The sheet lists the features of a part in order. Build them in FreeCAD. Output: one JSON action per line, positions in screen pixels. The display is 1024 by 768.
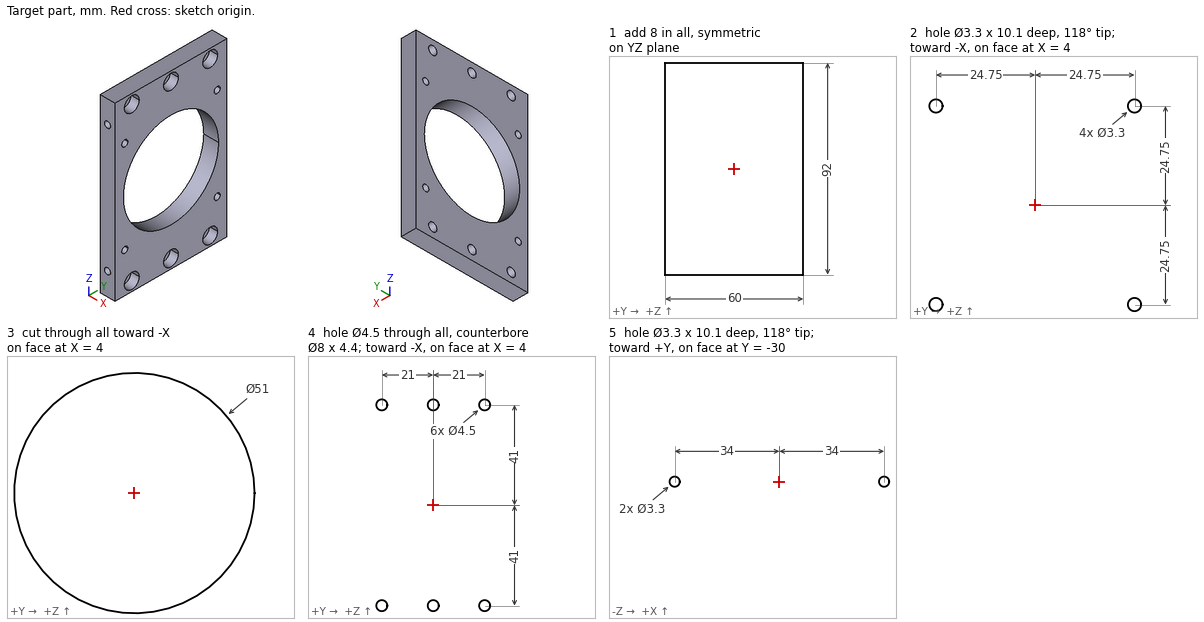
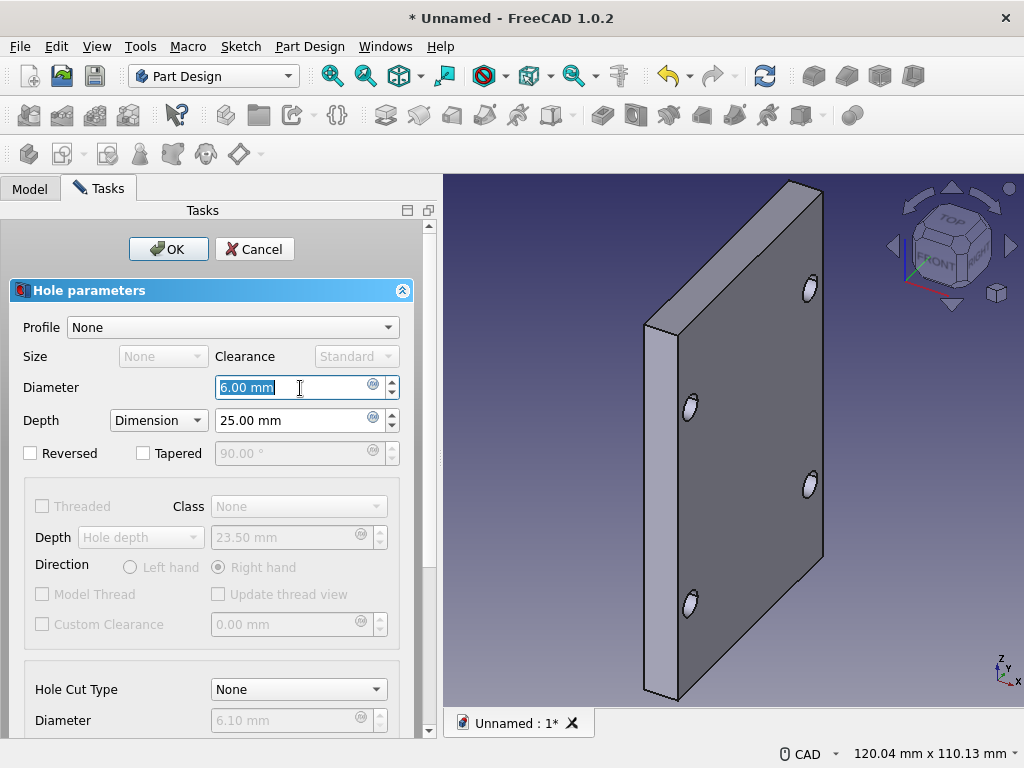
{"action": "type", "text": "3.3"}
{"action": "key", "text": "Tab"}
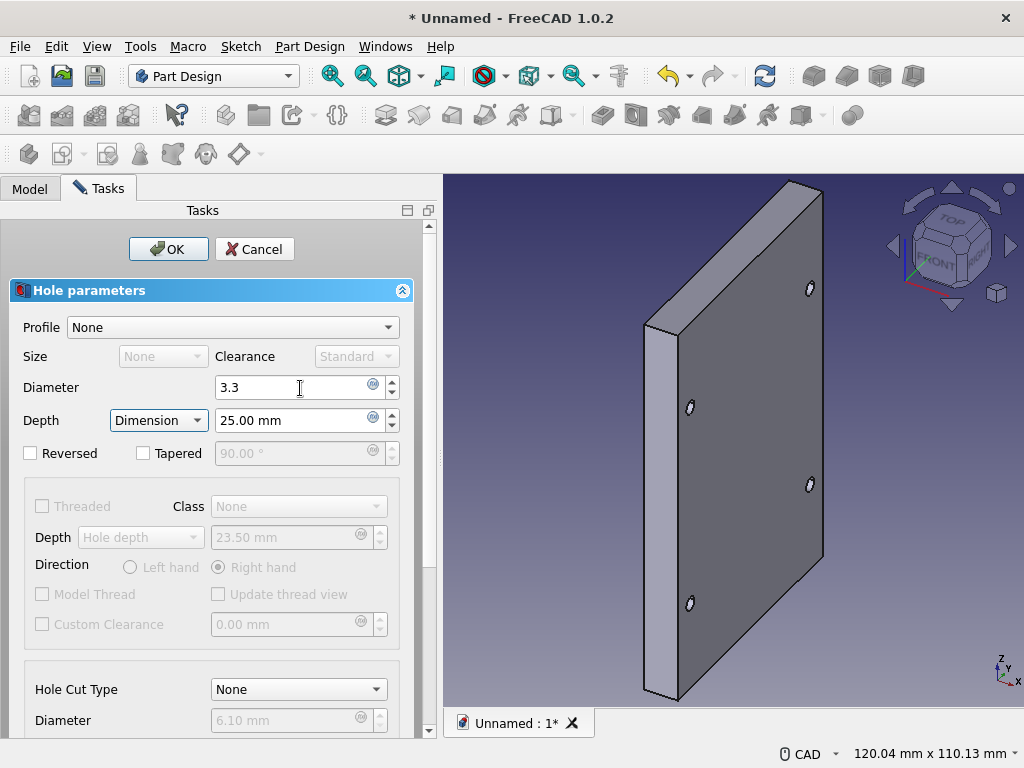
{"action": "triple_click", "coordinate": [300, 420]}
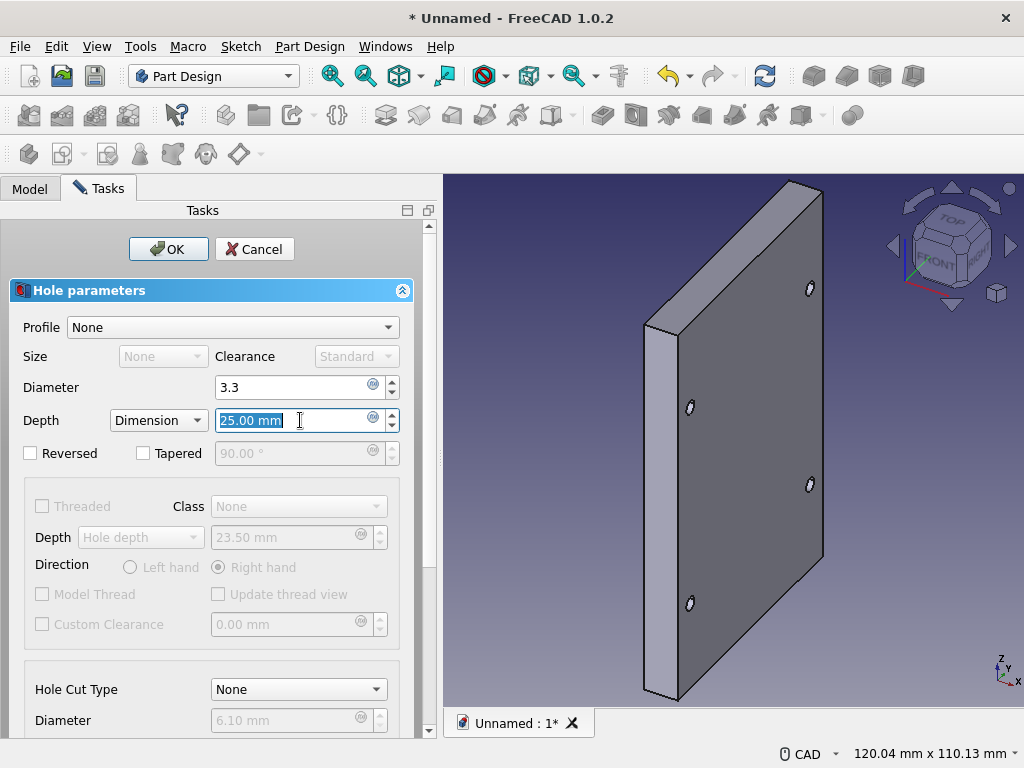
{"action": "type", "text": "10.1"}
{"action": "key", "text": "Tab"}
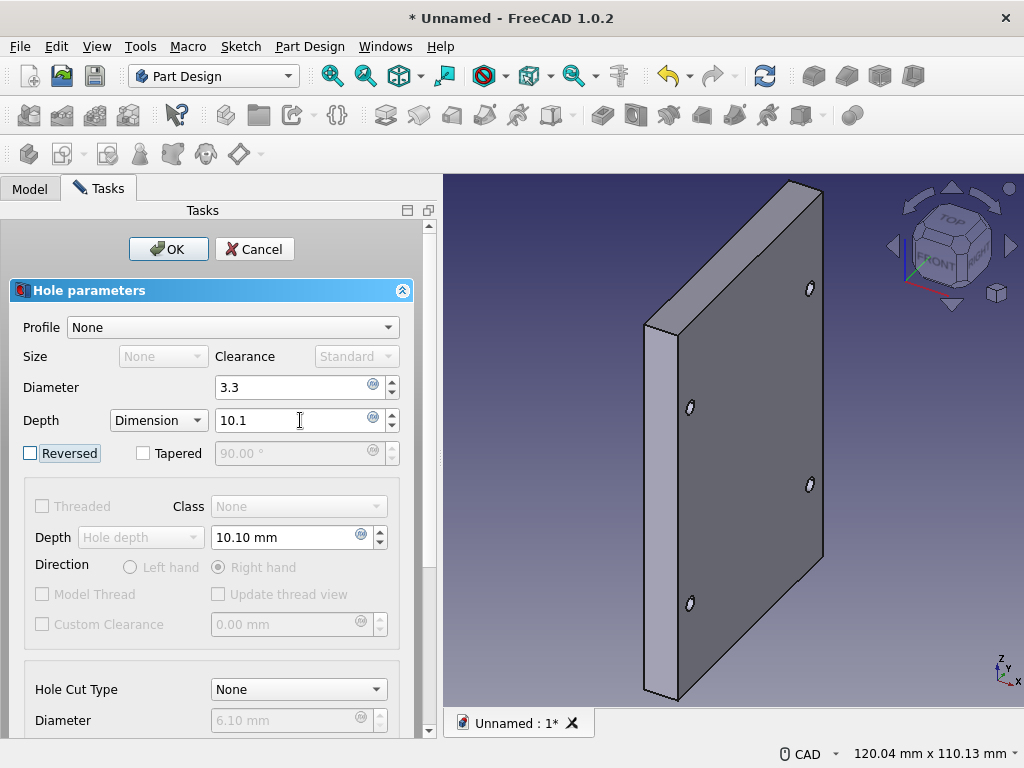
{"action": "left_click", "coordinate": [169, 249]}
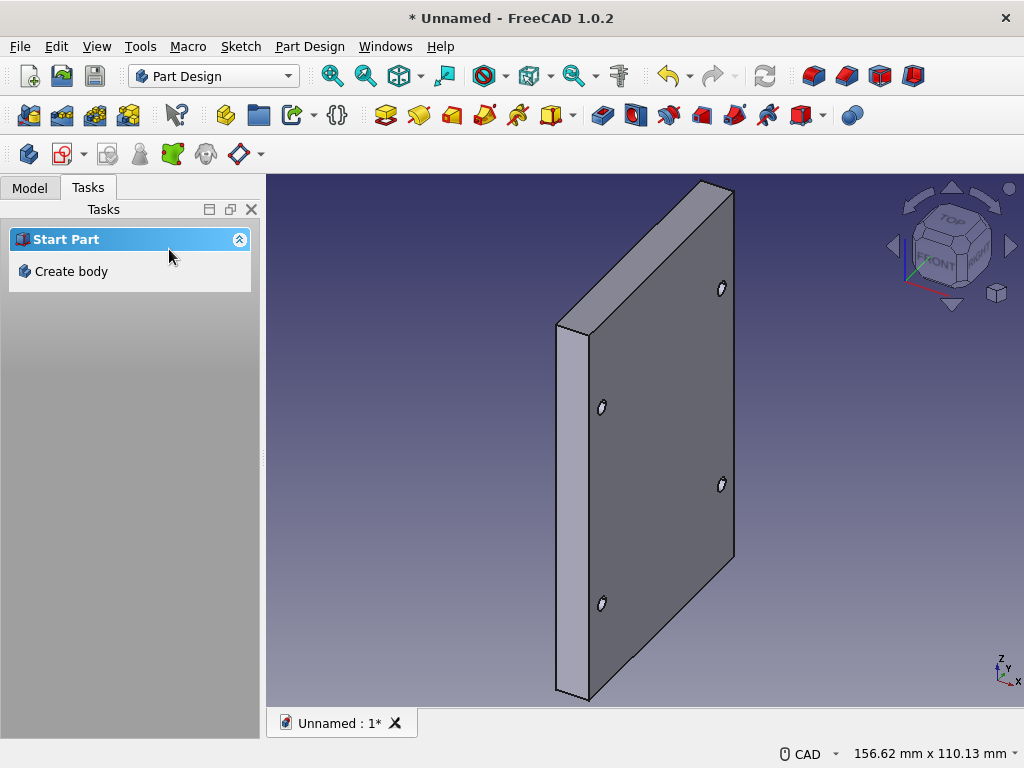
{"action": "left_click", "coordinate": [662, 445]}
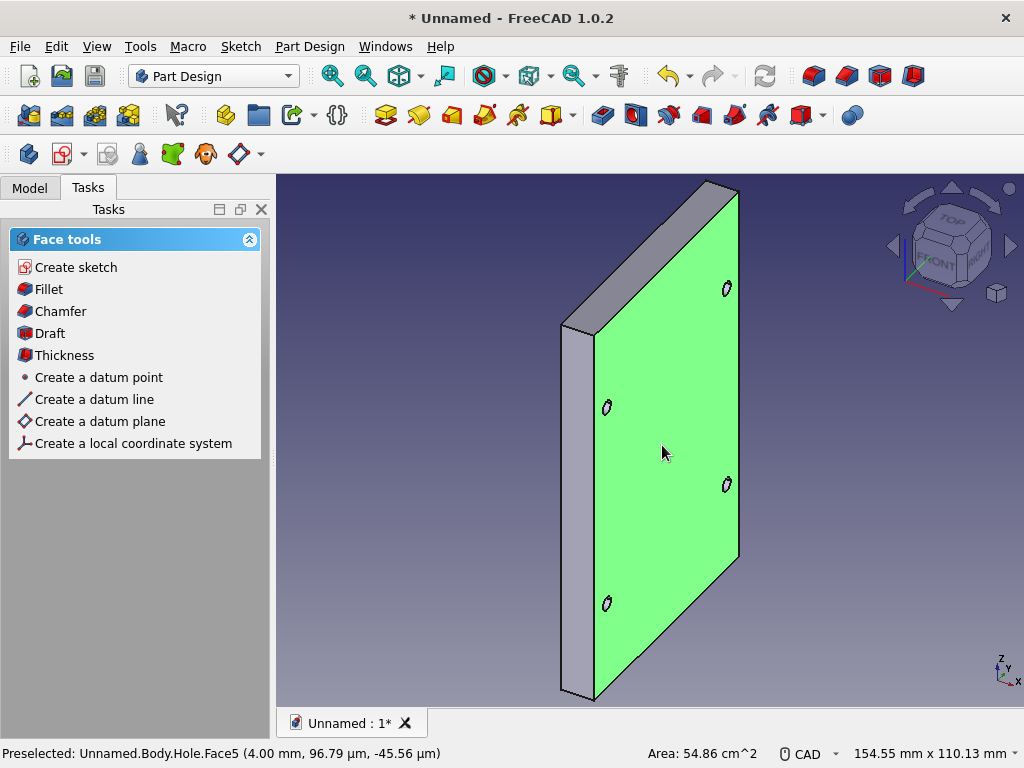
{"action": "left_click", "coordinate": [62, 154]}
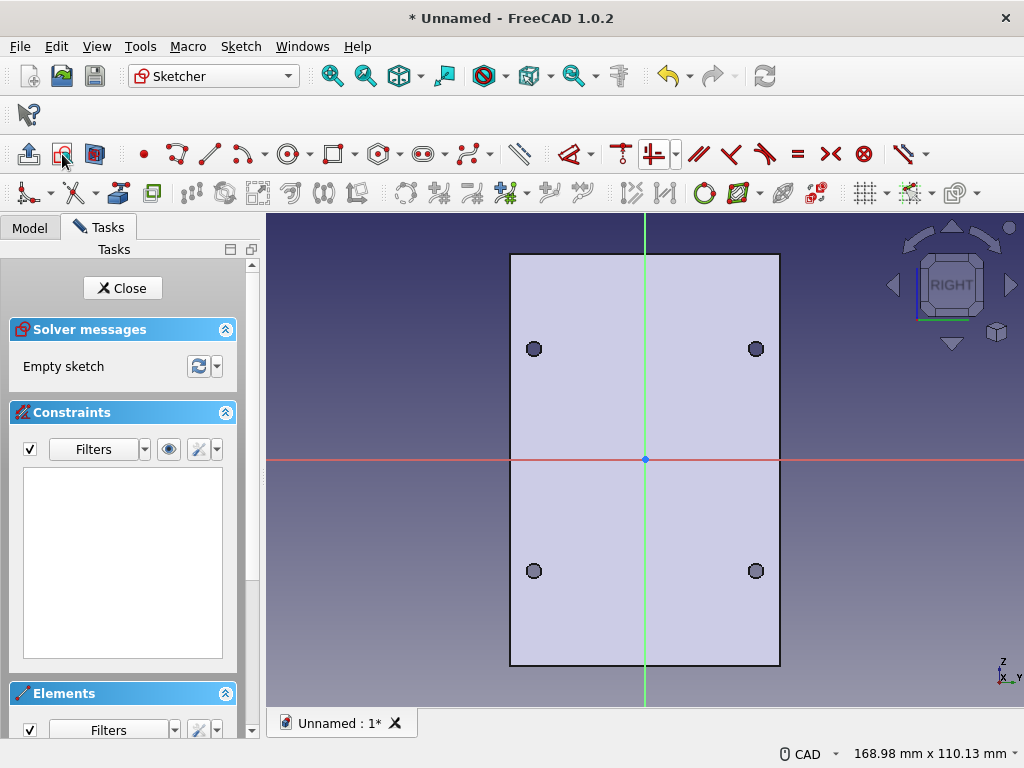
{"action": "scroll", "coordinate": [784, 460], "scroll_direction": "up", "scroll_amount": 2}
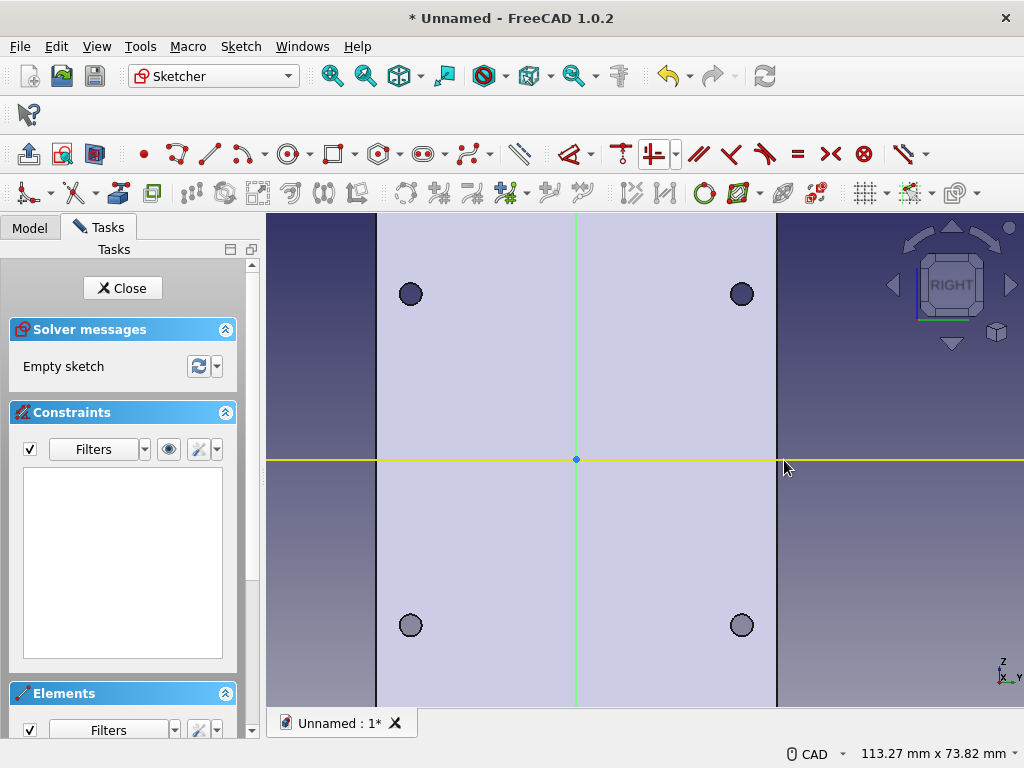
{"action": "left_click", "coordinate": [288, 154]}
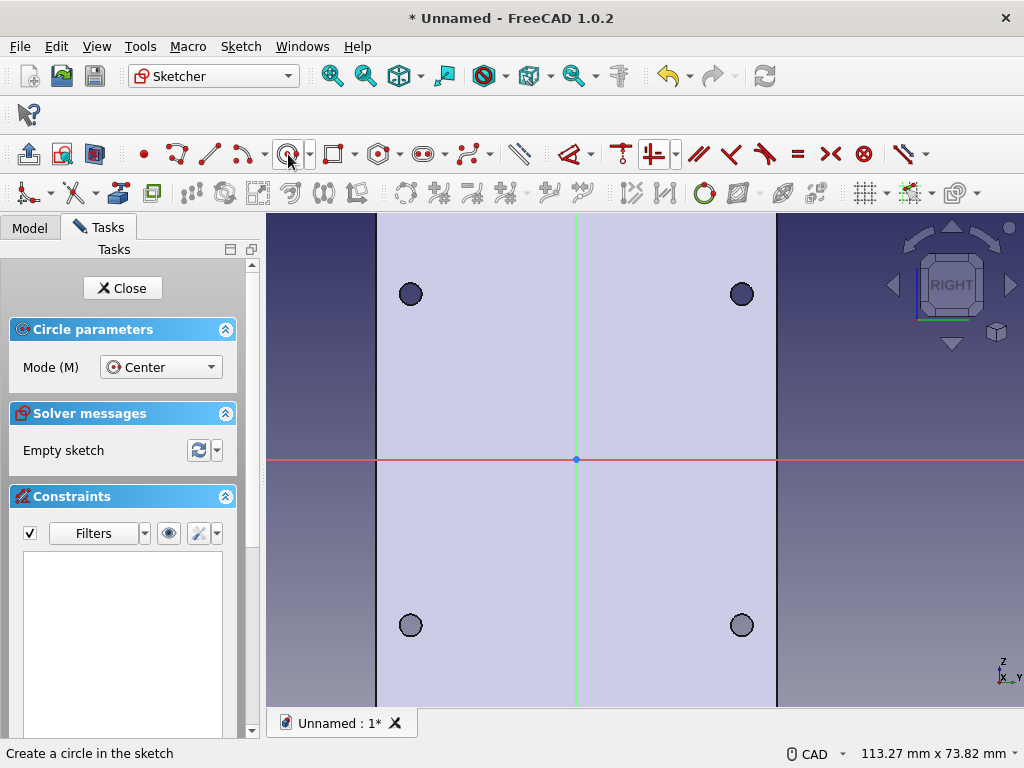
{"action": "left_click", "coordinate": [576, 460]}
{"action": "left_click", "coordinate": [697, 339]}
{"action": "key", "text": "Escape"}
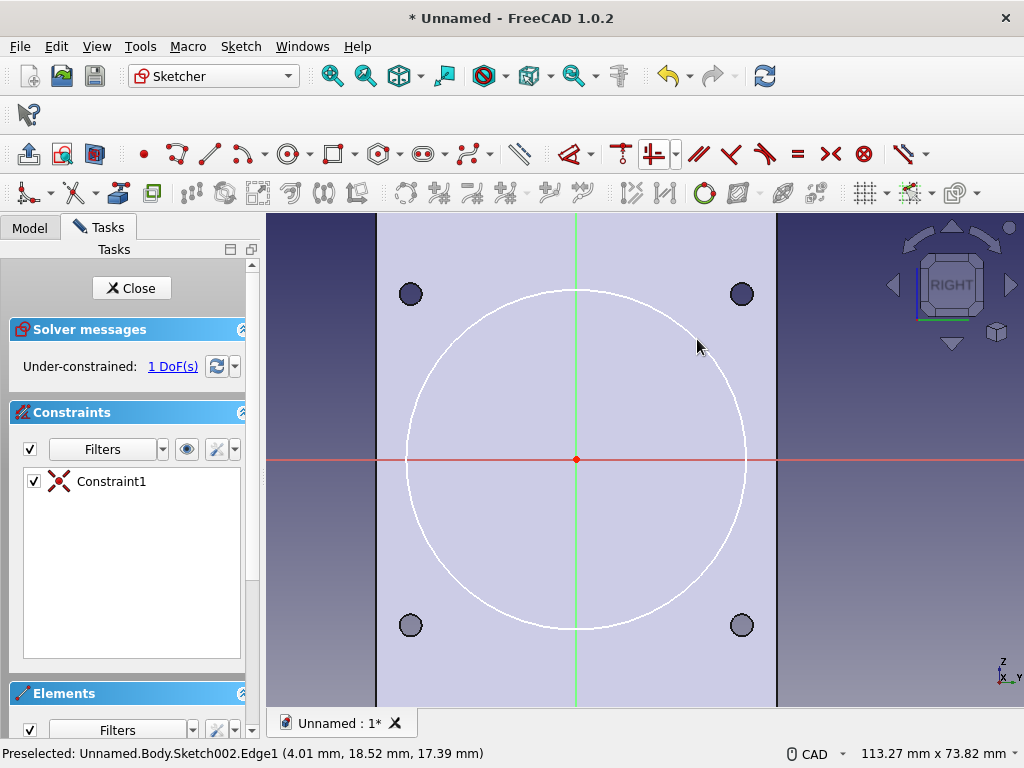
{"action": "left_click", "coordinate": [568, 154]}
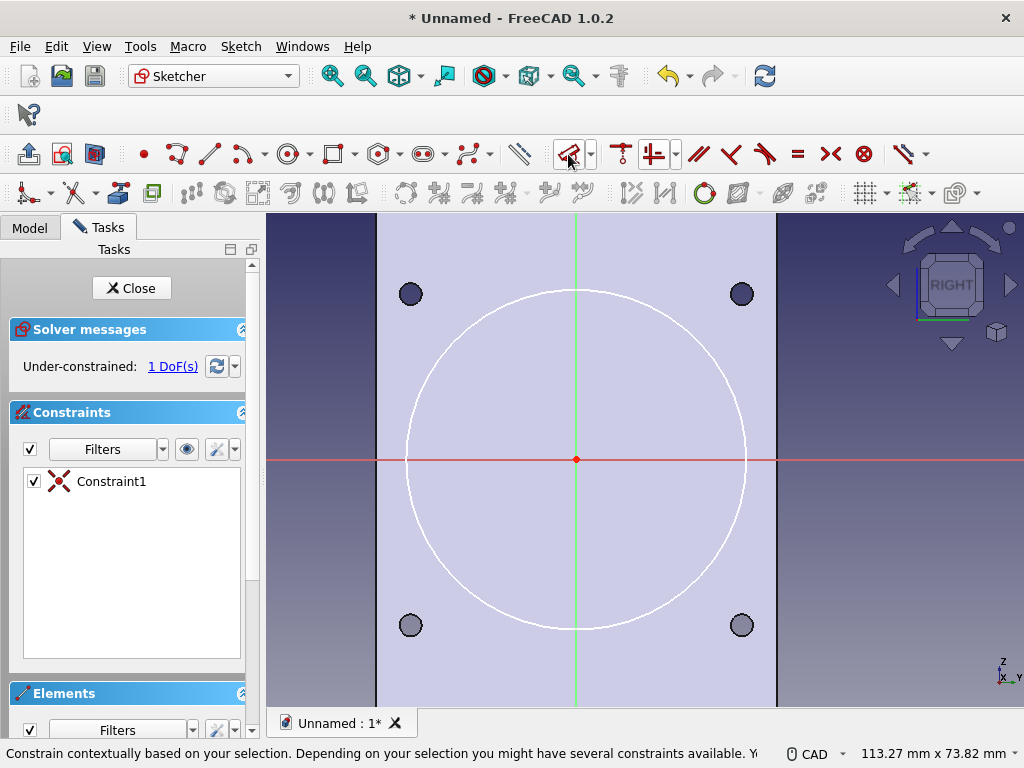
{"action": "left_click", "coordinate": [696, 339]}
{"action": "left_click", "coordinate": [719, 316]}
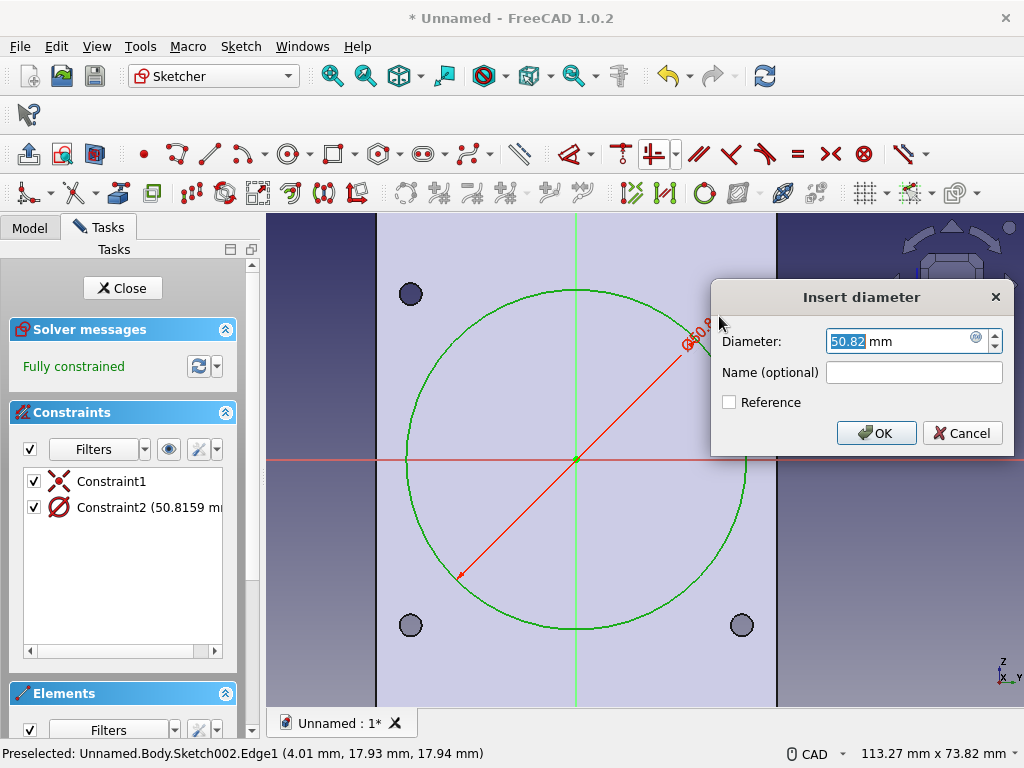
{"action": "type", "text": "51"}
{"action": "key", "text": "Return"}
{"action": "key", "text": "Escape"}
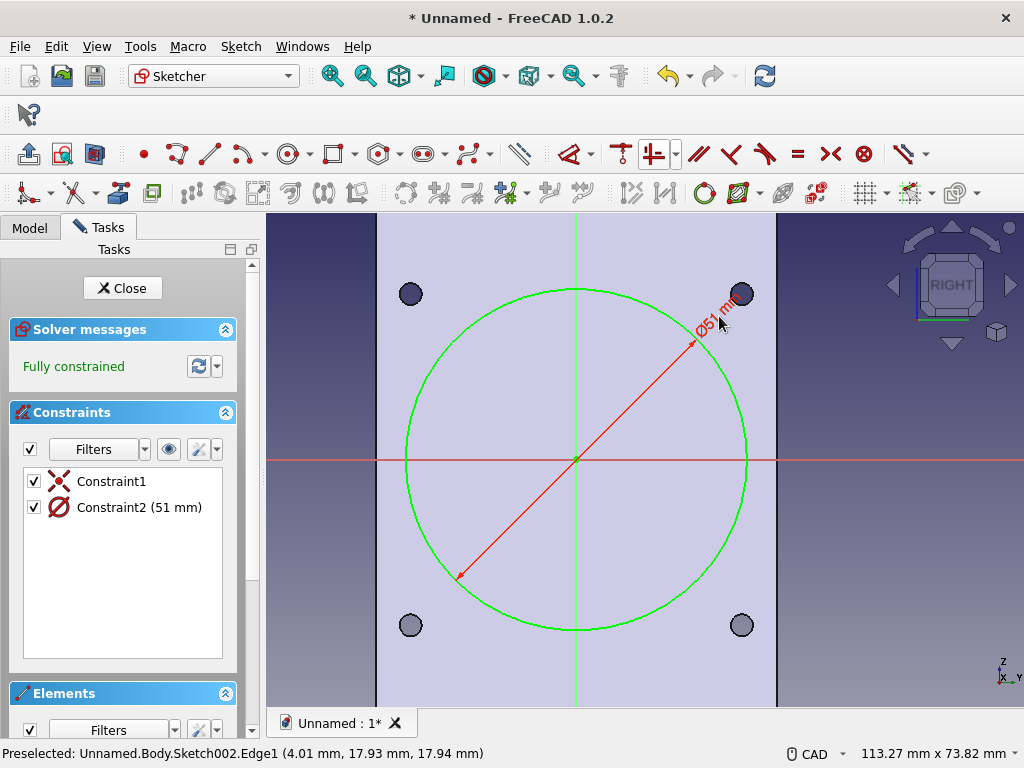
{"action": "left_click", "coordinate": [123, 288]}